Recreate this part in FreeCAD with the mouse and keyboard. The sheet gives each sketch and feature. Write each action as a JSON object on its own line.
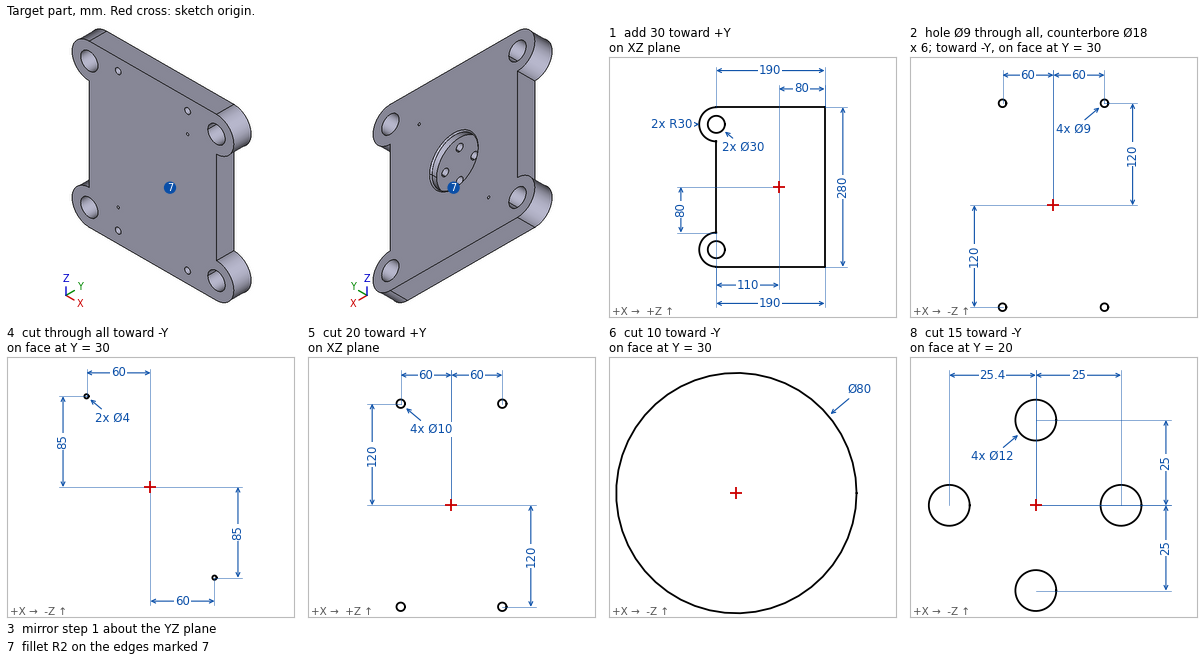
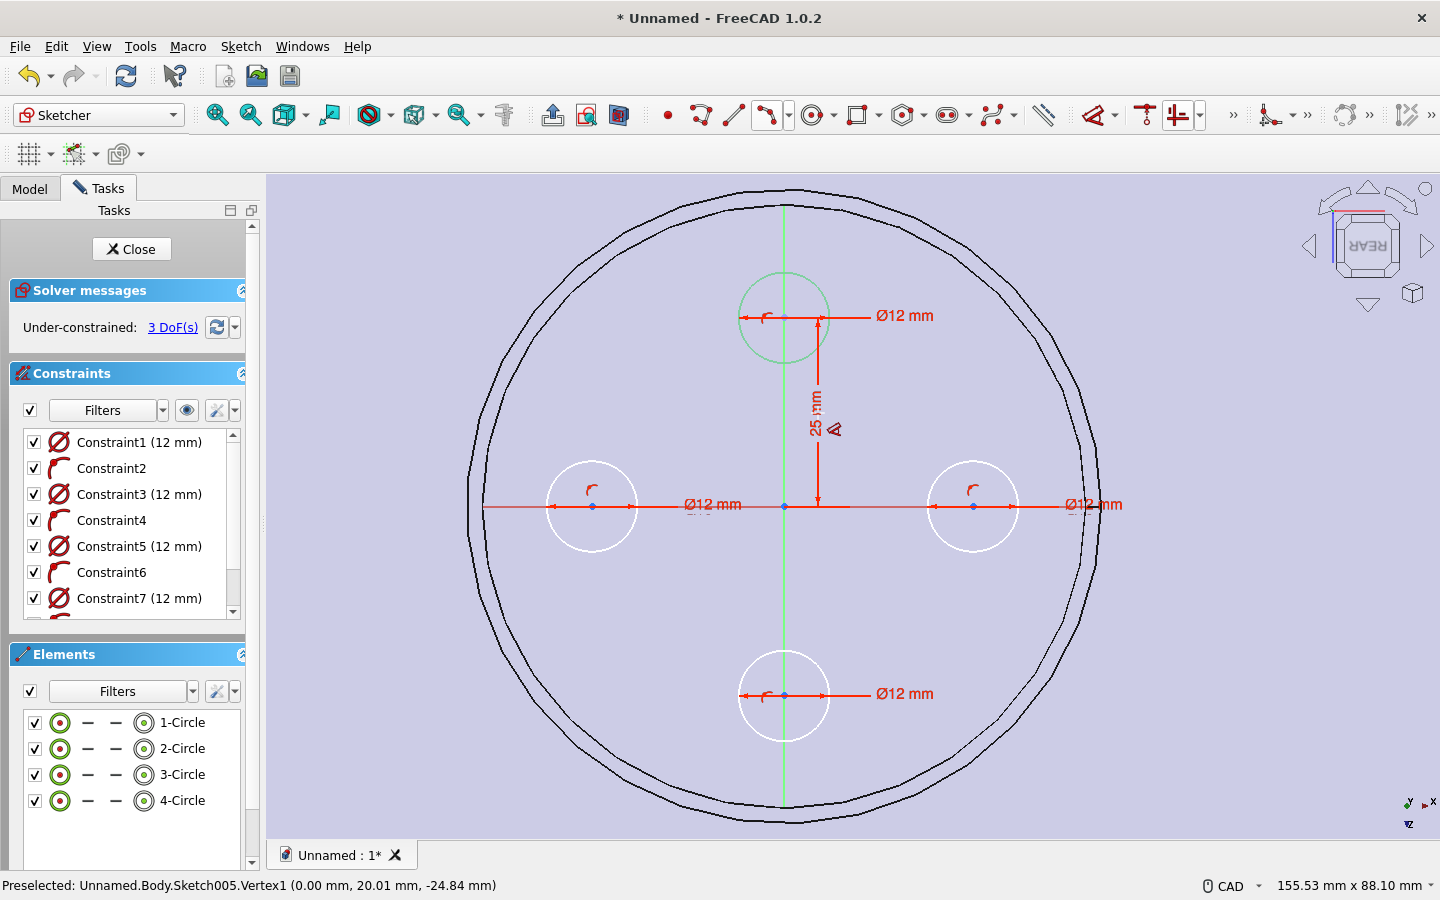
{"action": "left_click", "coordinate": [973, 506]}
{"action": "left_click", "coordinate": [879, 540]}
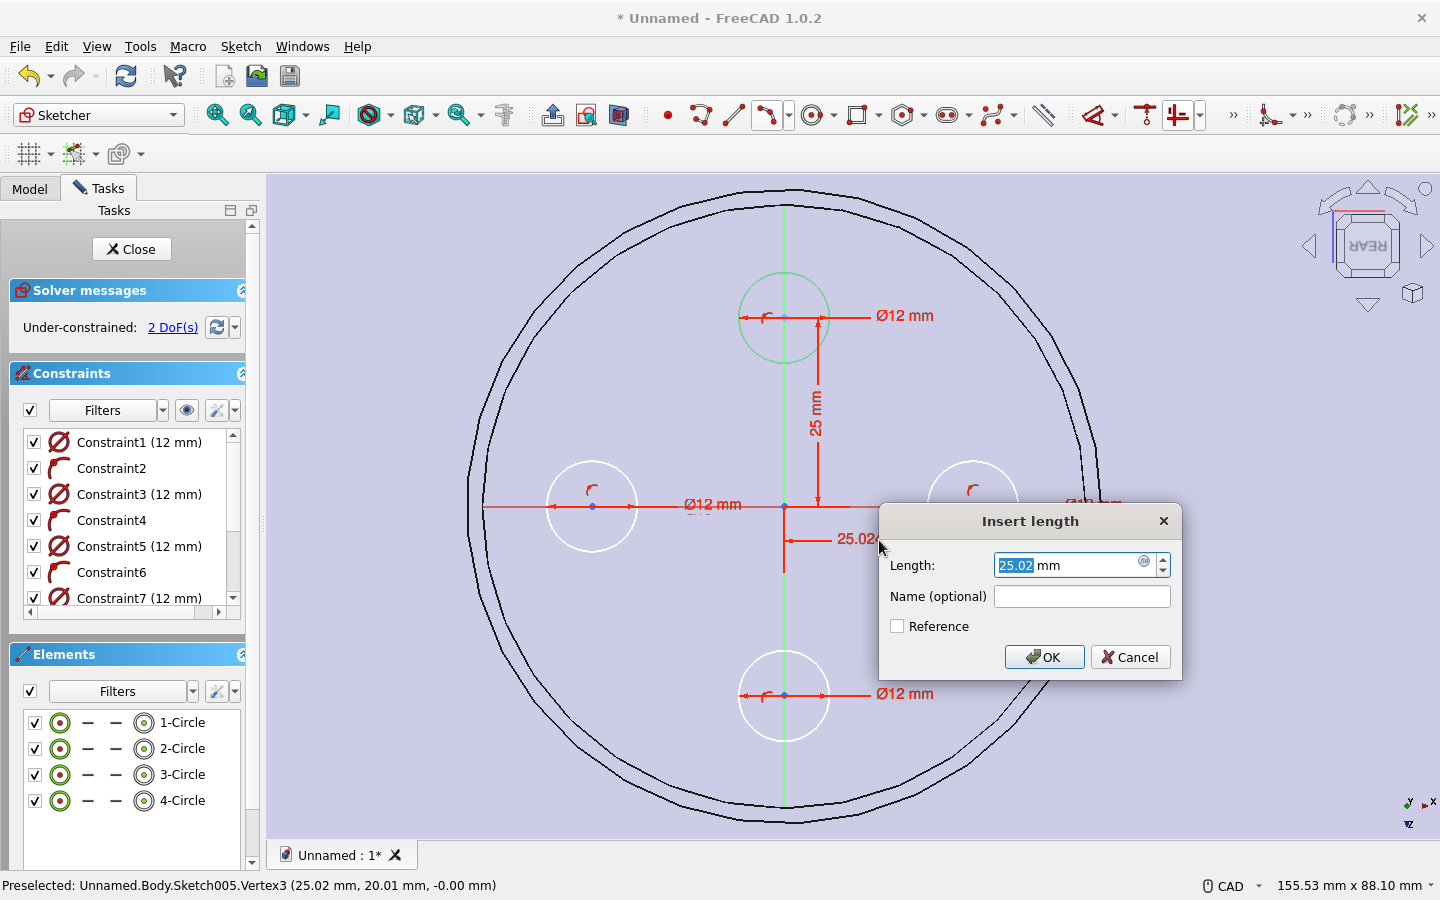
{"action": "type", "text": "25"}
{"action": "key", "text": "Return"}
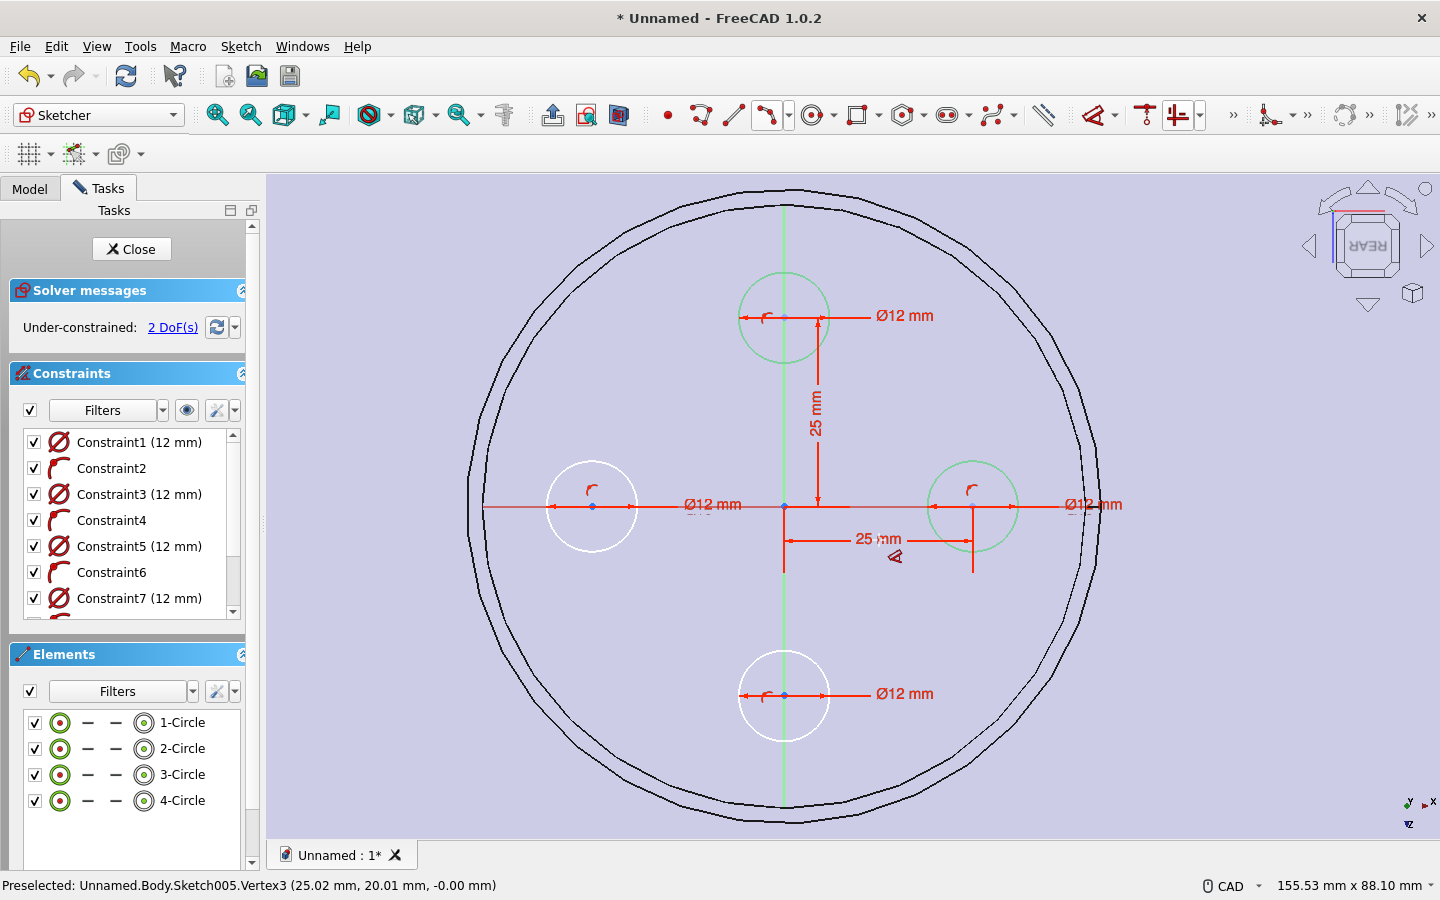
{"action": "left_click", "coordinate": [784, 696]}
{"action": "left_click", "coordinate": [818, 601]}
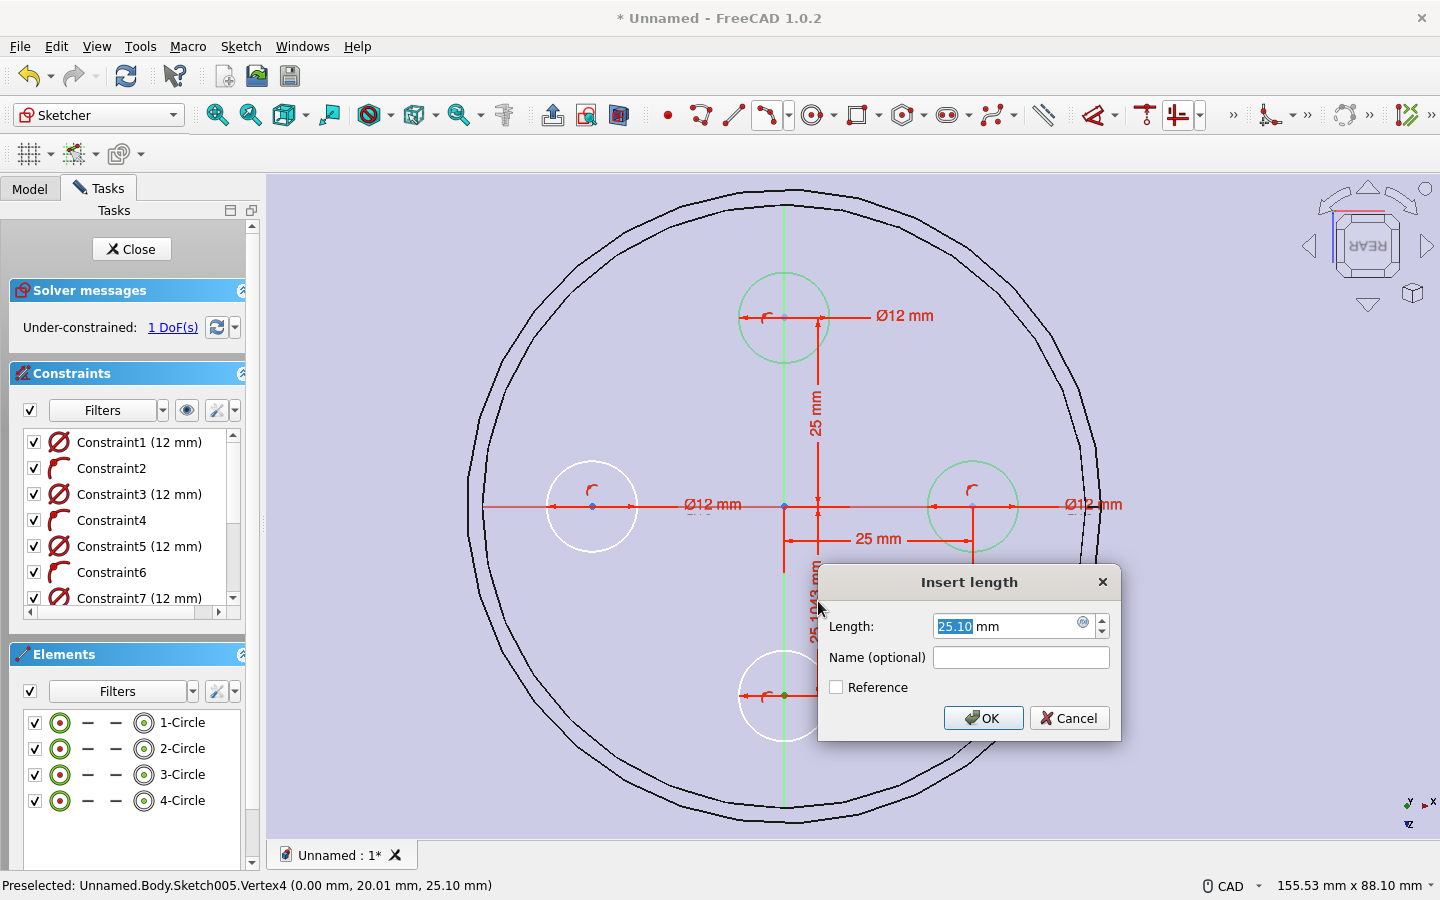
{"action": "type", "text": "25"}
{"action": "key", "text": "Return"}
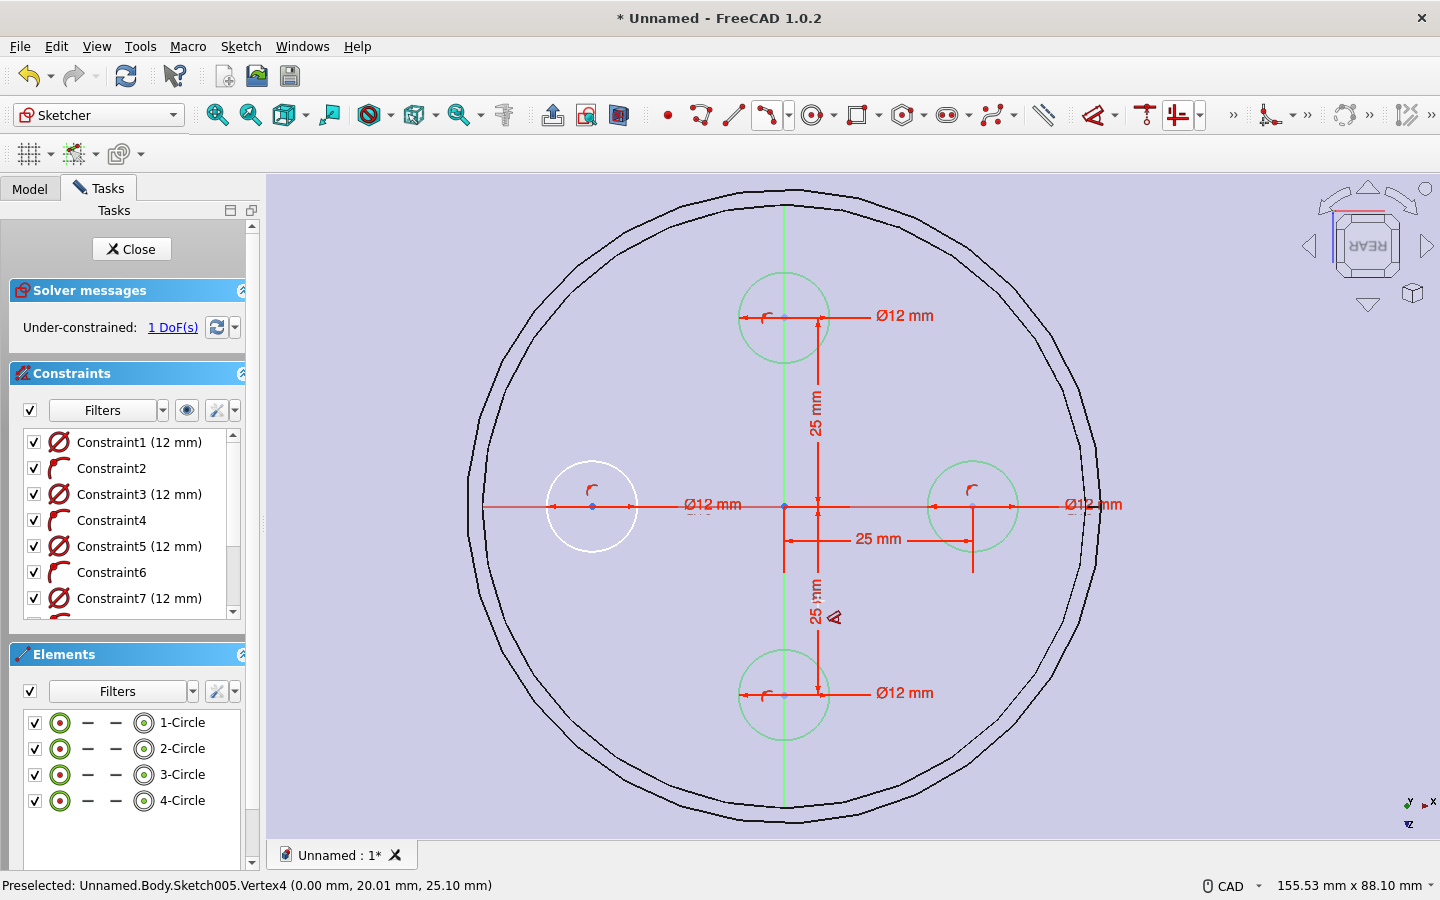
{"action": "left_click", "coordinate": [592, 506]}
{"action": "left_click", "coordinate": [688, 540]}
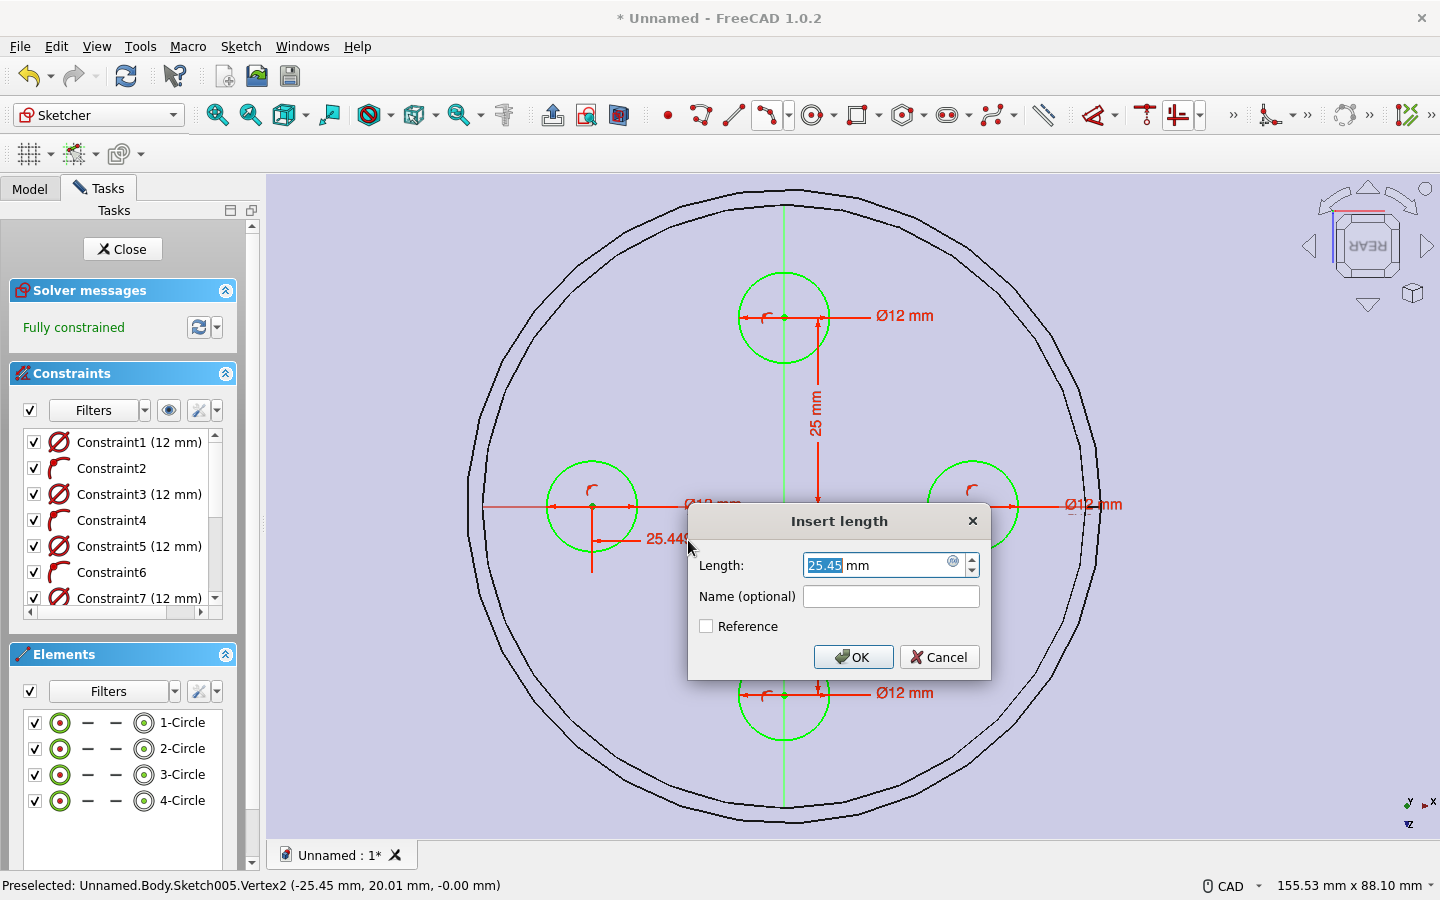
{"action": "type", "text": "25.4"}
{"action": "key", "text": "Return"}
{"action": "key", "text": "Escape"}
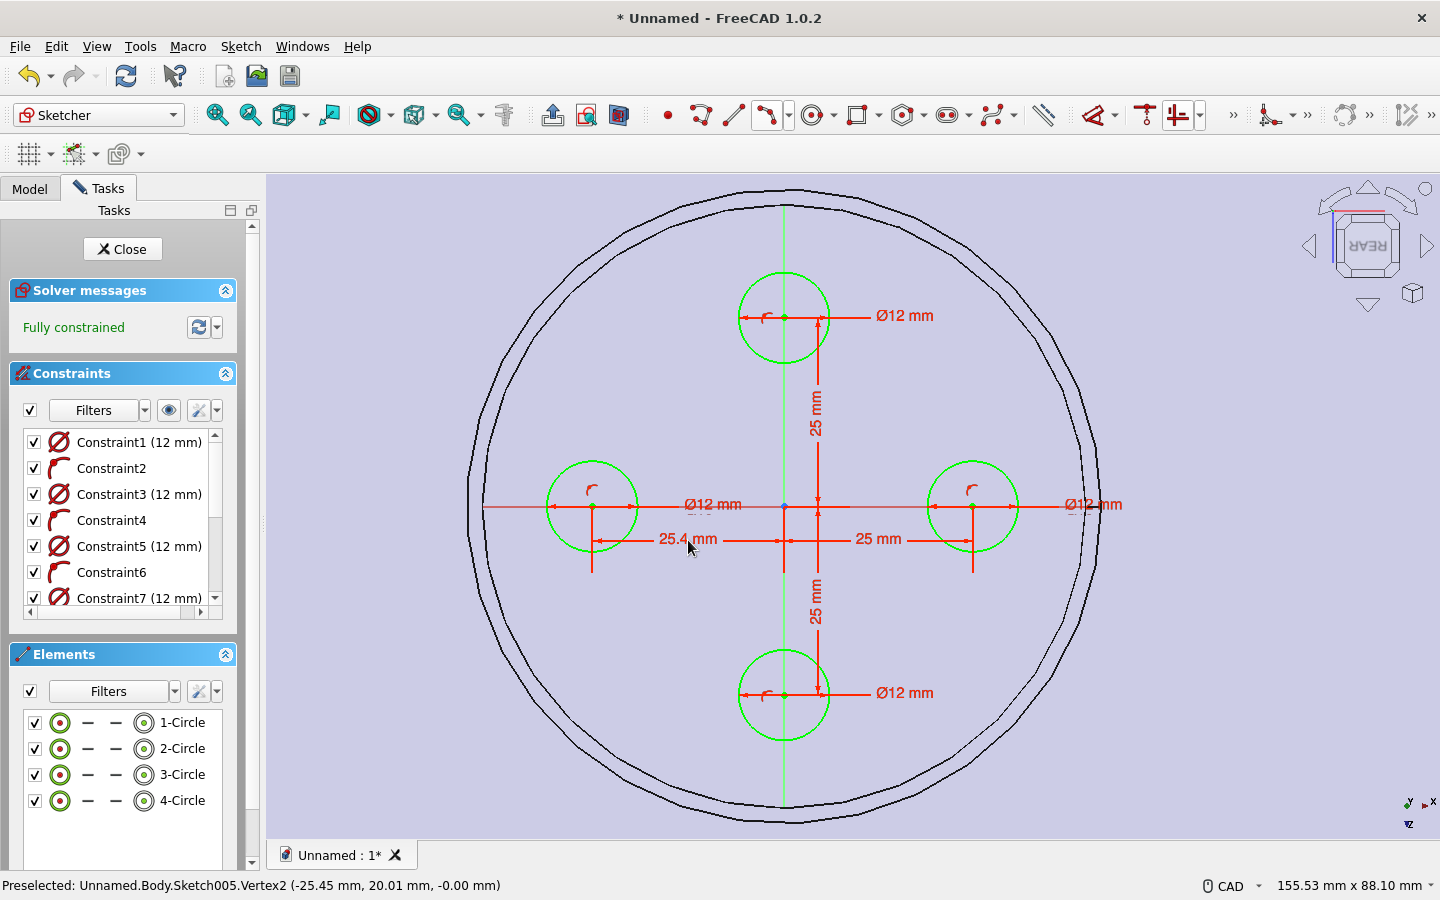
{"action": "left_click", "coordinate": [123, 249]}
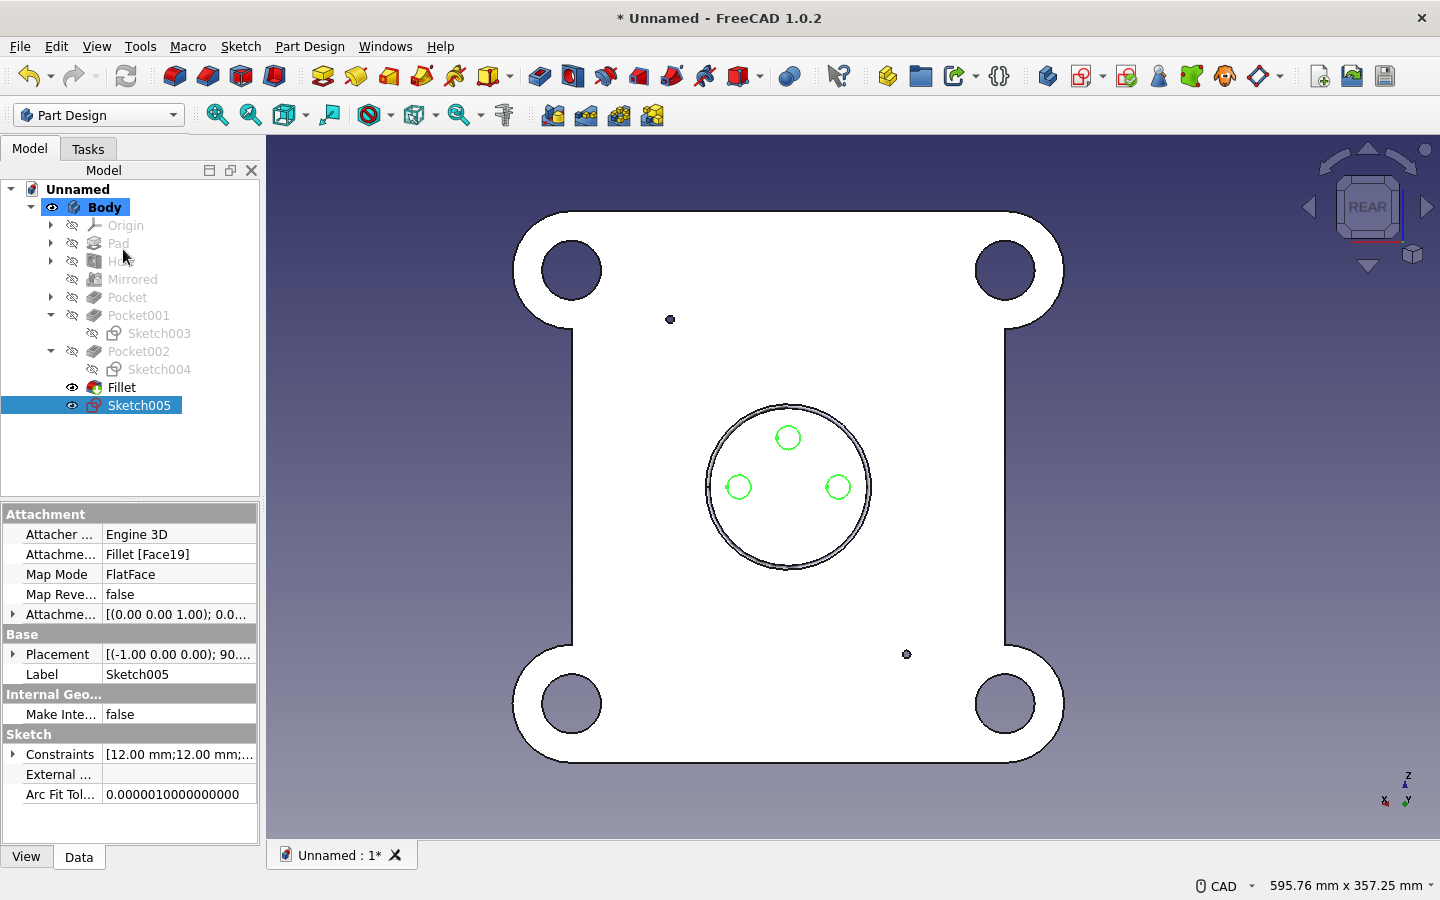
{"action": "left_click", "coordinate": [540, 76]}